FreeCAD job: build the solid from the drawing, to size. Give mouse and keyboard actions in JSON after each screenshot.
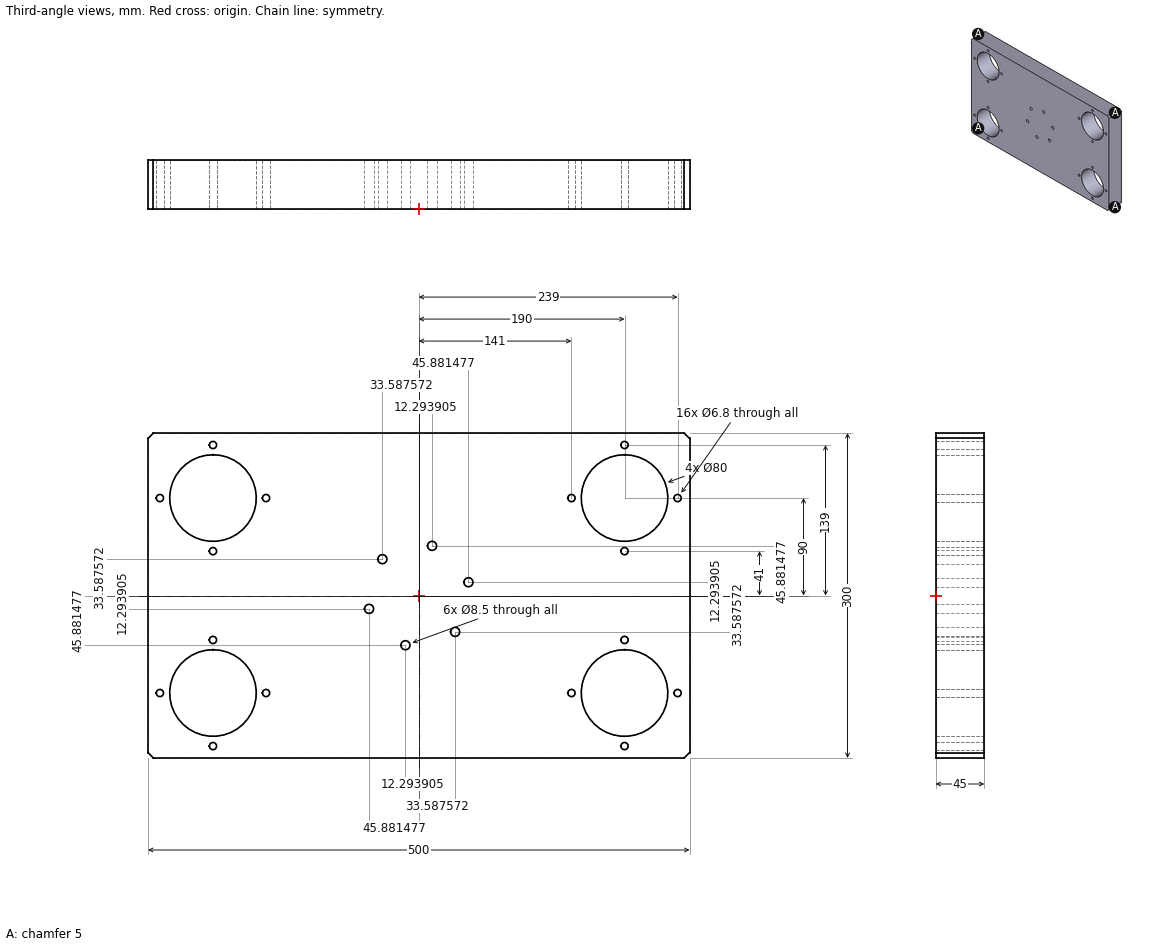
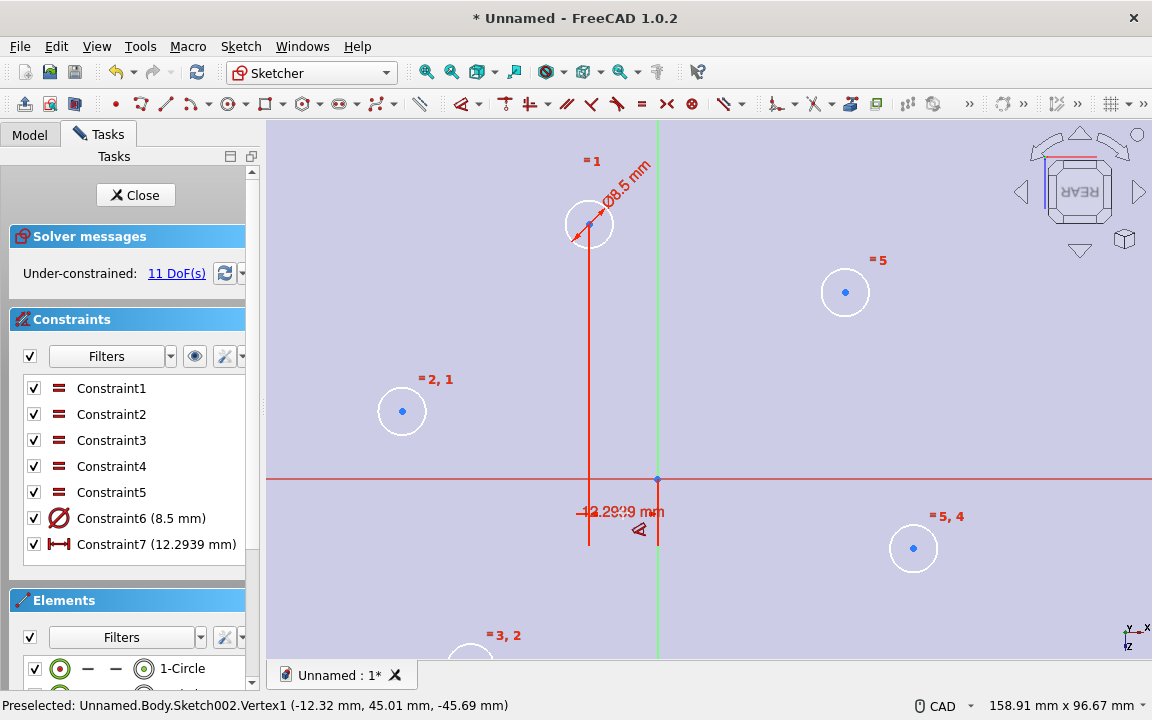
{"action": "left_click", "coordinate": [589, 224]}
{"action": "left_click", "coordinate": [555, 352]}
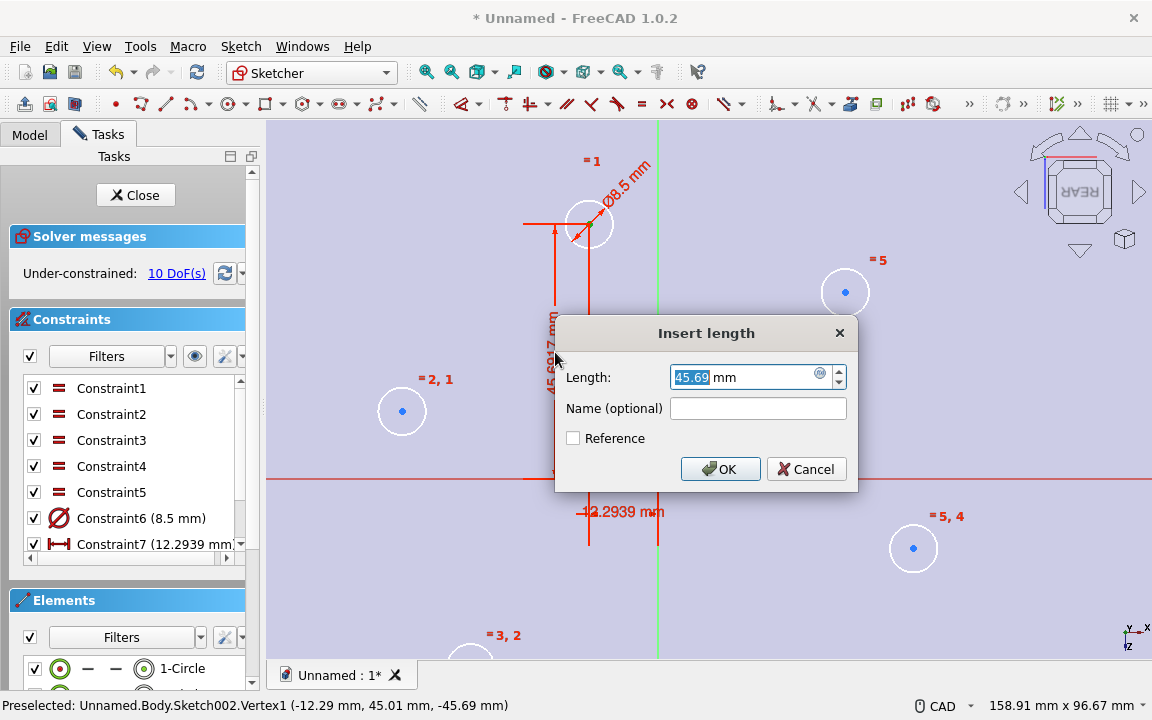
{"action": "type", "text": "45.881477"}
{"action": "key", "text": "Return"}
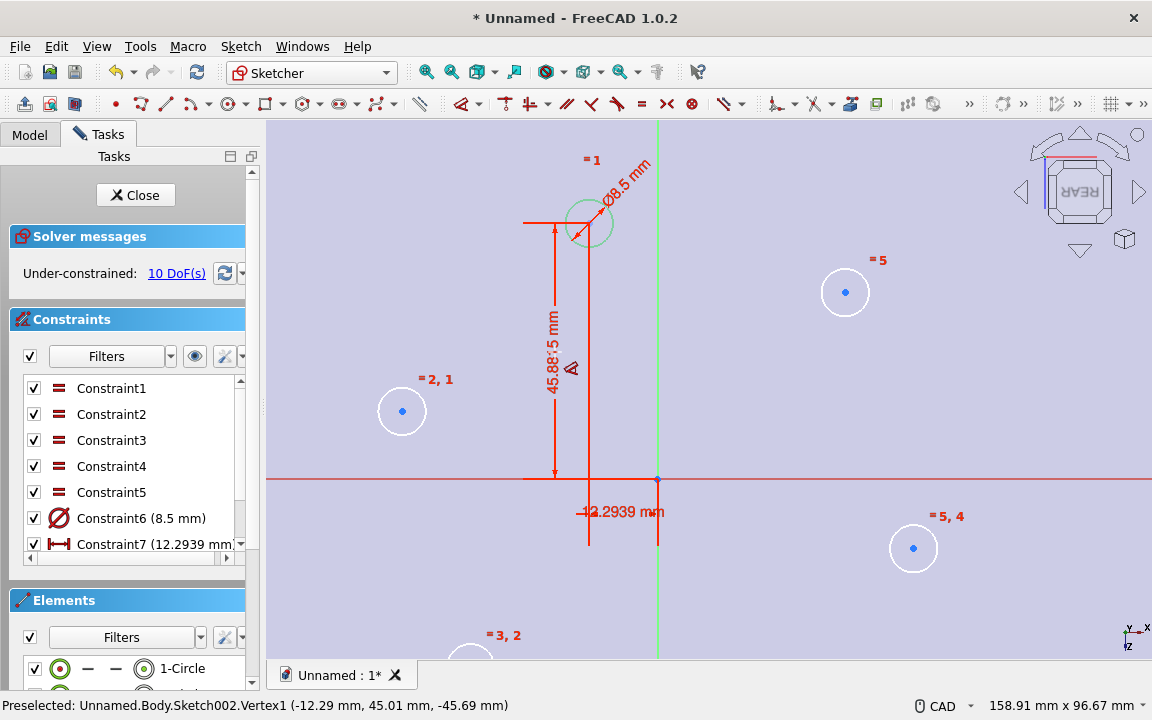
{"action": "left_click", "coordinate": [402, 411]}
{"action": "left_click", "coordinate": [530, 377]}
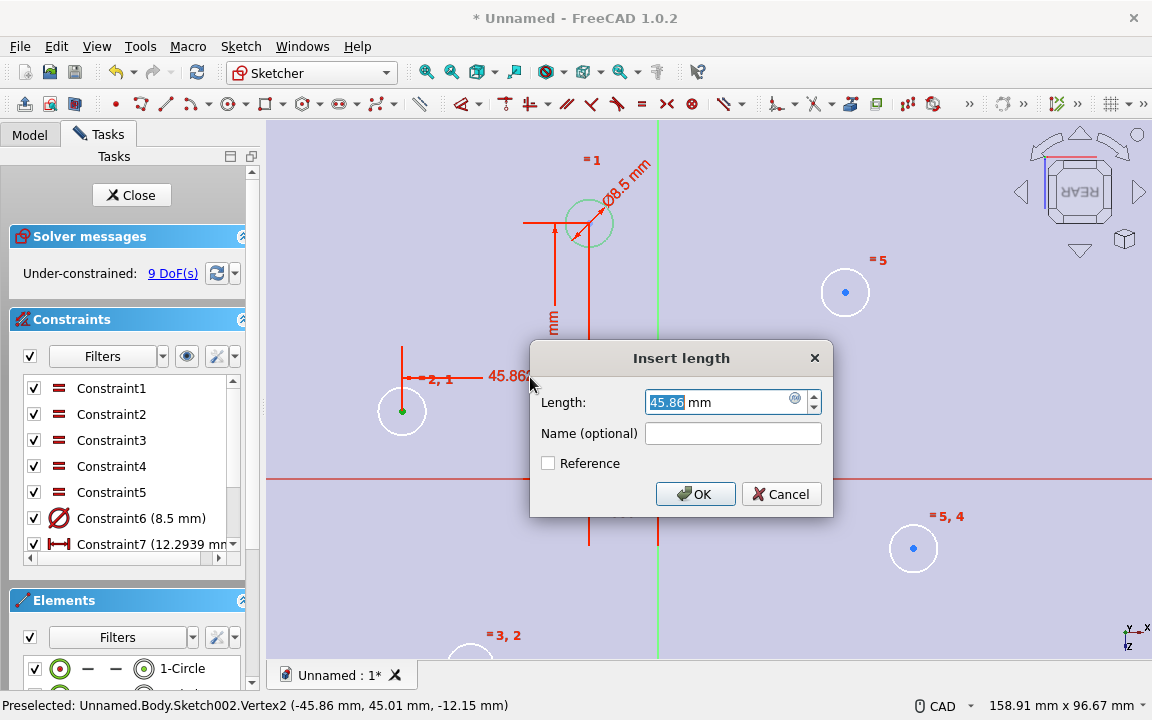
{"action": "type", "text": "45.881477"}
{"action": "key", "text": "Return"}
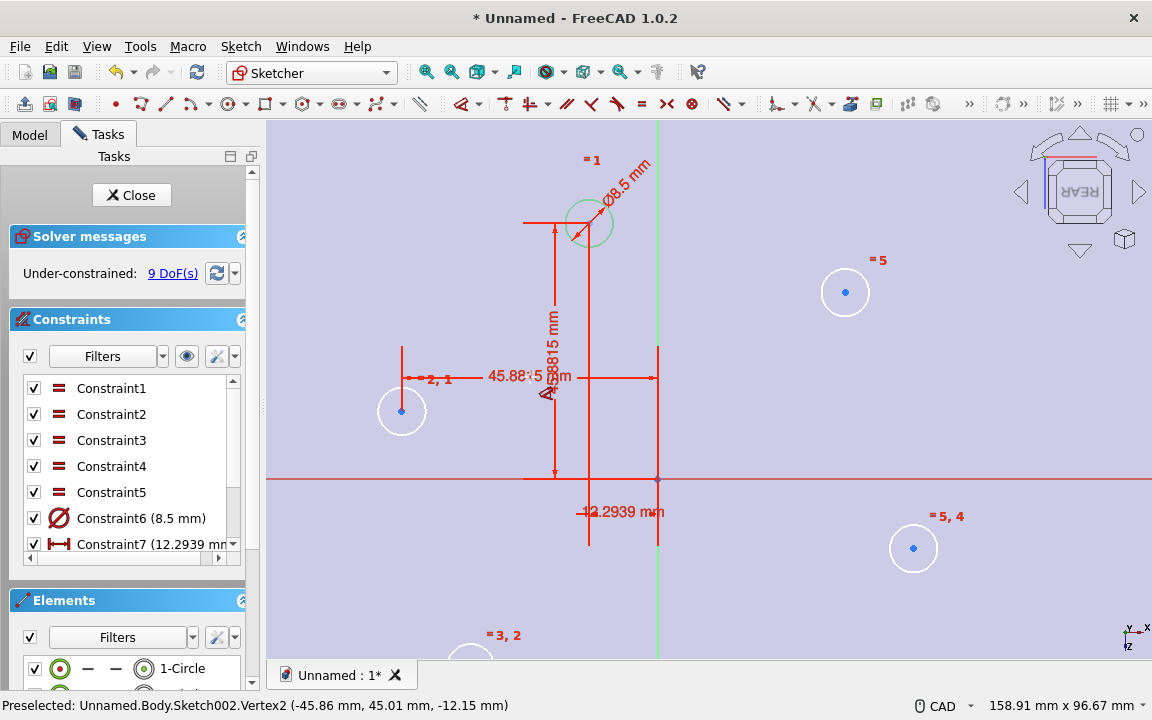
{"action": "left_click", "coordinate": [402, 411]}
{"action": "left_click", "coordinate": [368, 445]}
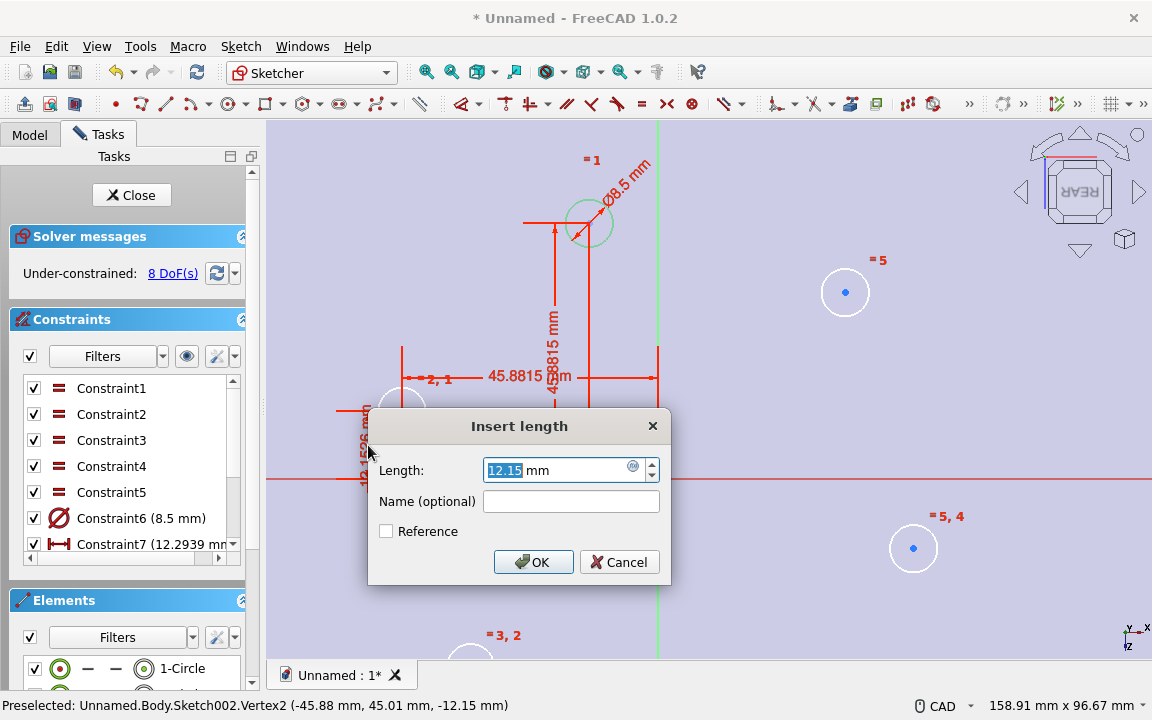
{"action": "type", "text": "12.293905"}
{"action": "key", "text": "Return"}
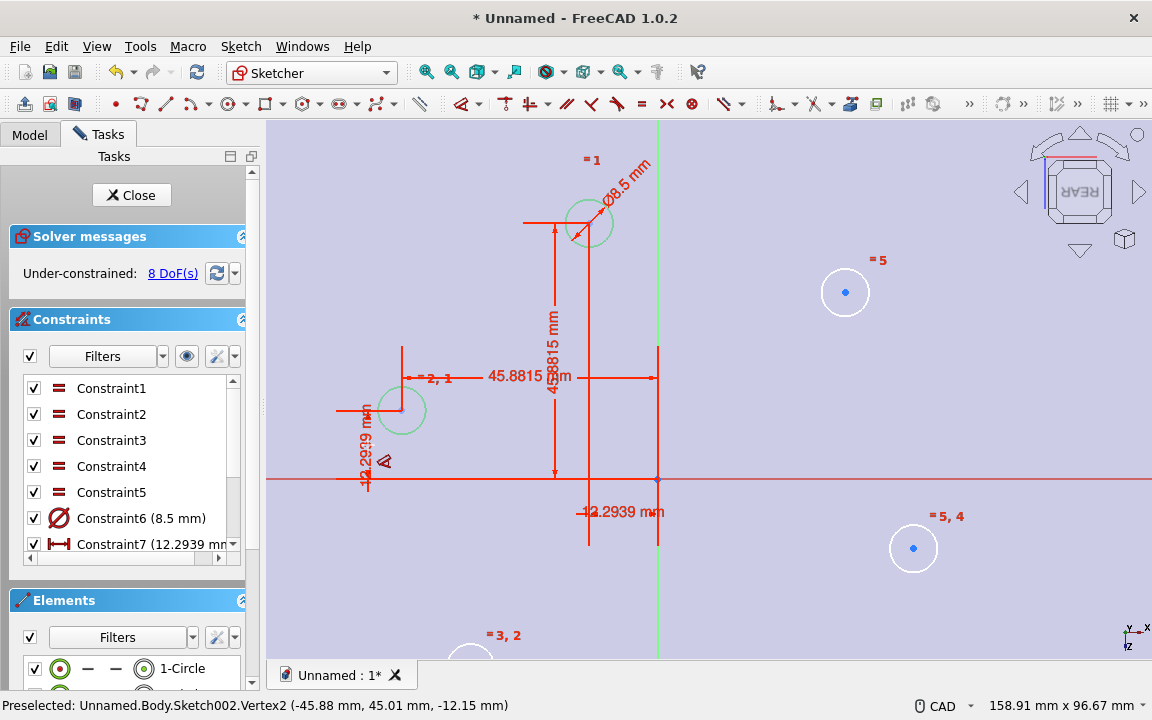
{"action": "scroll", "coordinate": [605, 207], "scroll_direction": "down", "scroll_amount": 2}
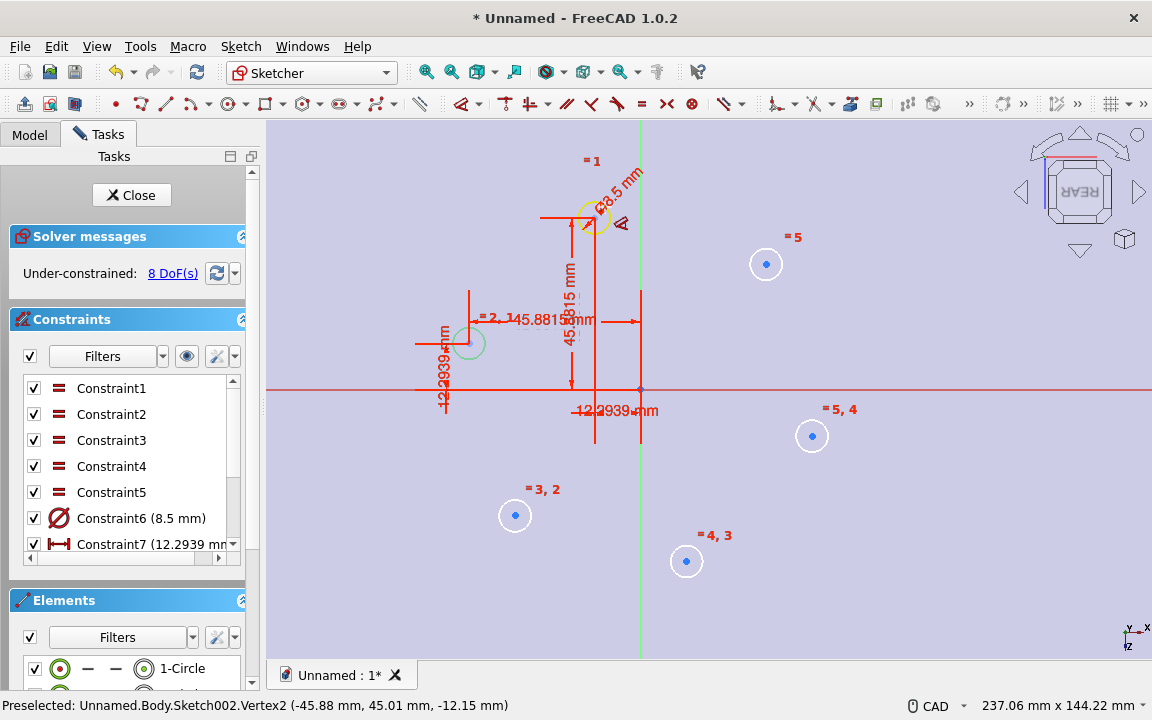
{"action": "left_click", "coordinate": [515, 516]}
{"action": "left_click", "coordinate": [578, 550]}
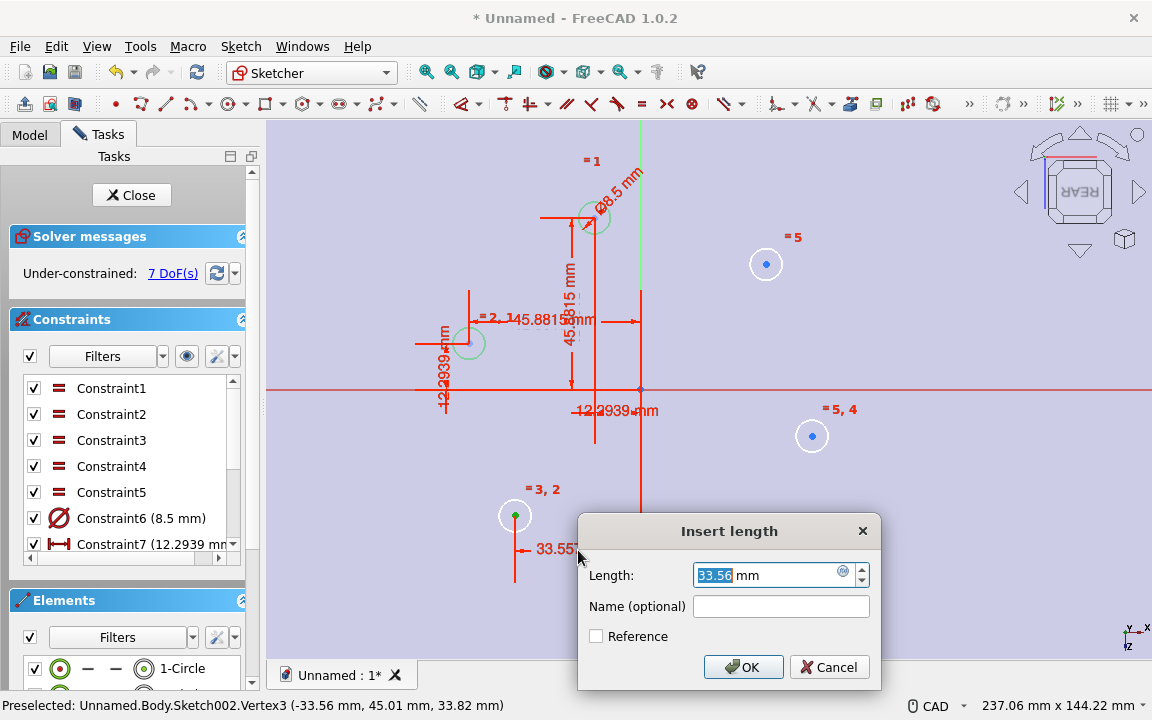
{"action": "type", "text": "33.587572"}
{"action": "key", "text": "Return"}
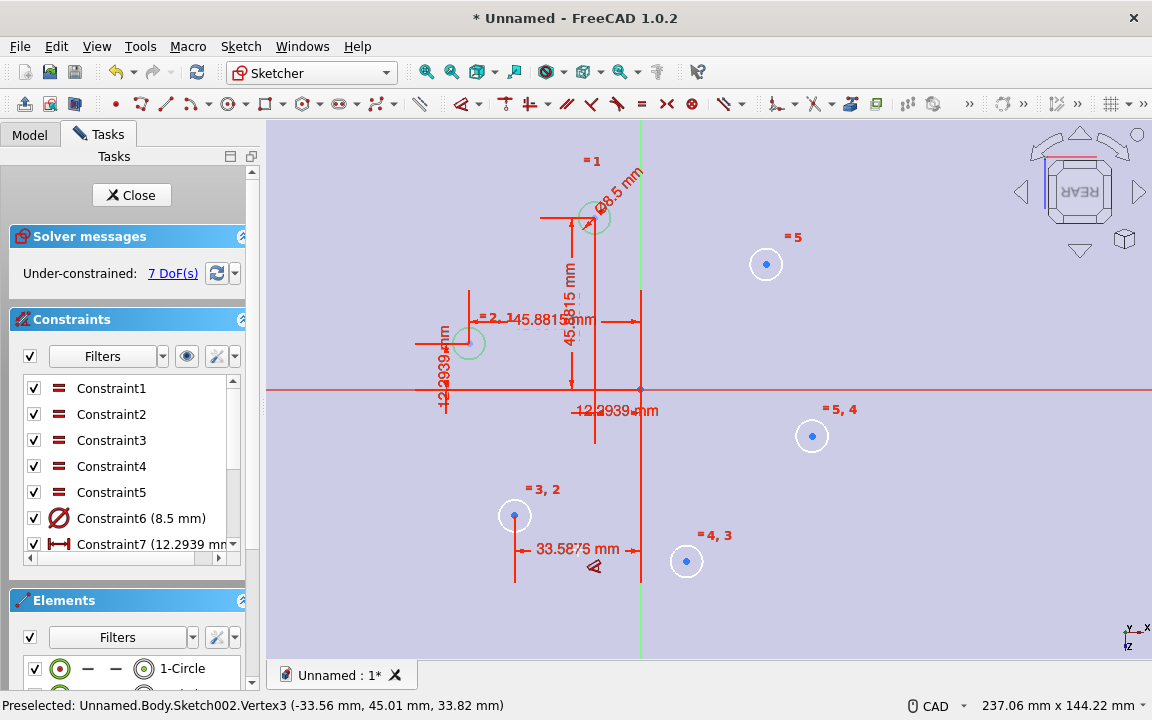
{"action": "left_click", "coordinate": [515, 516]}
{"action": "left_click", "coordinate": [481, 453]}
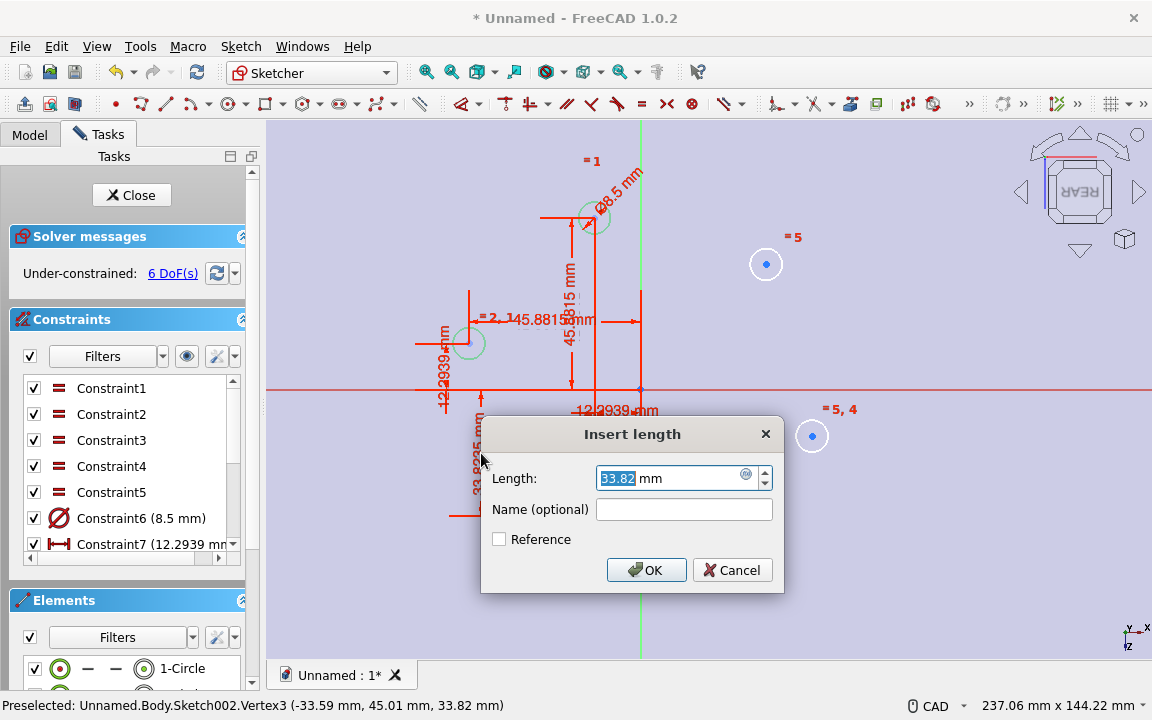
{"action": "type", "text": "33.587572"}
{"action": "key", "text": "Return"}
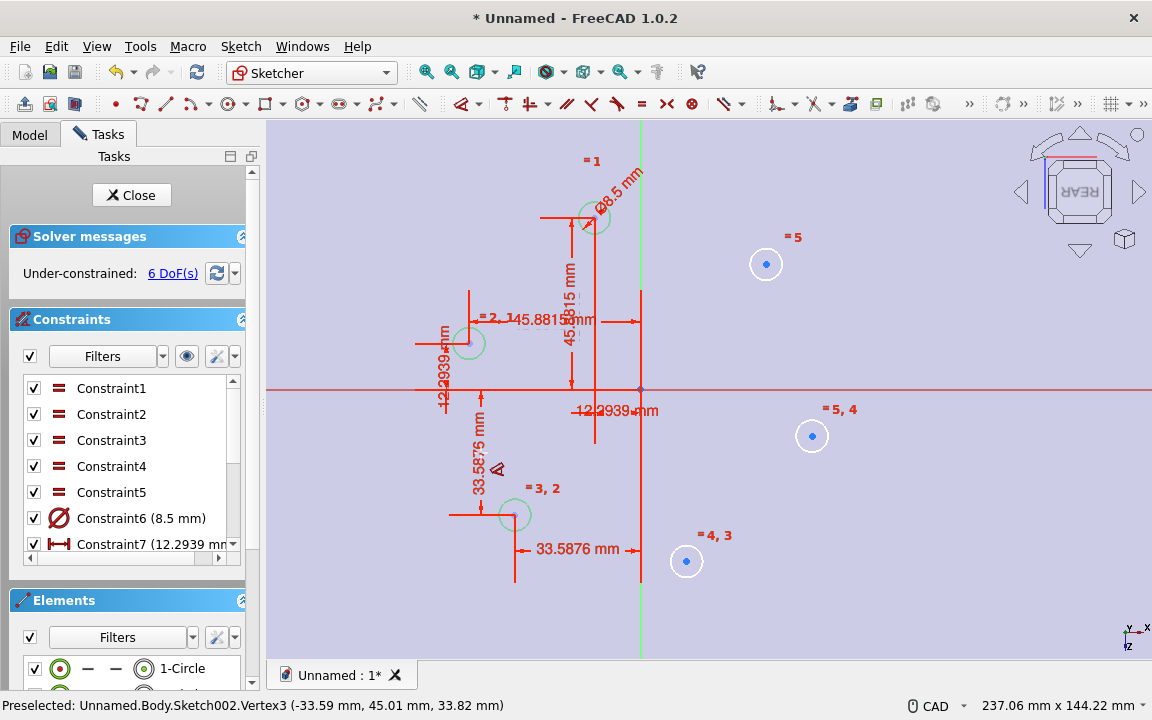
{"action": "left_click", "coordinate": [687, 561]}
{"action": "left_click", "coordinate": [664, 595]}